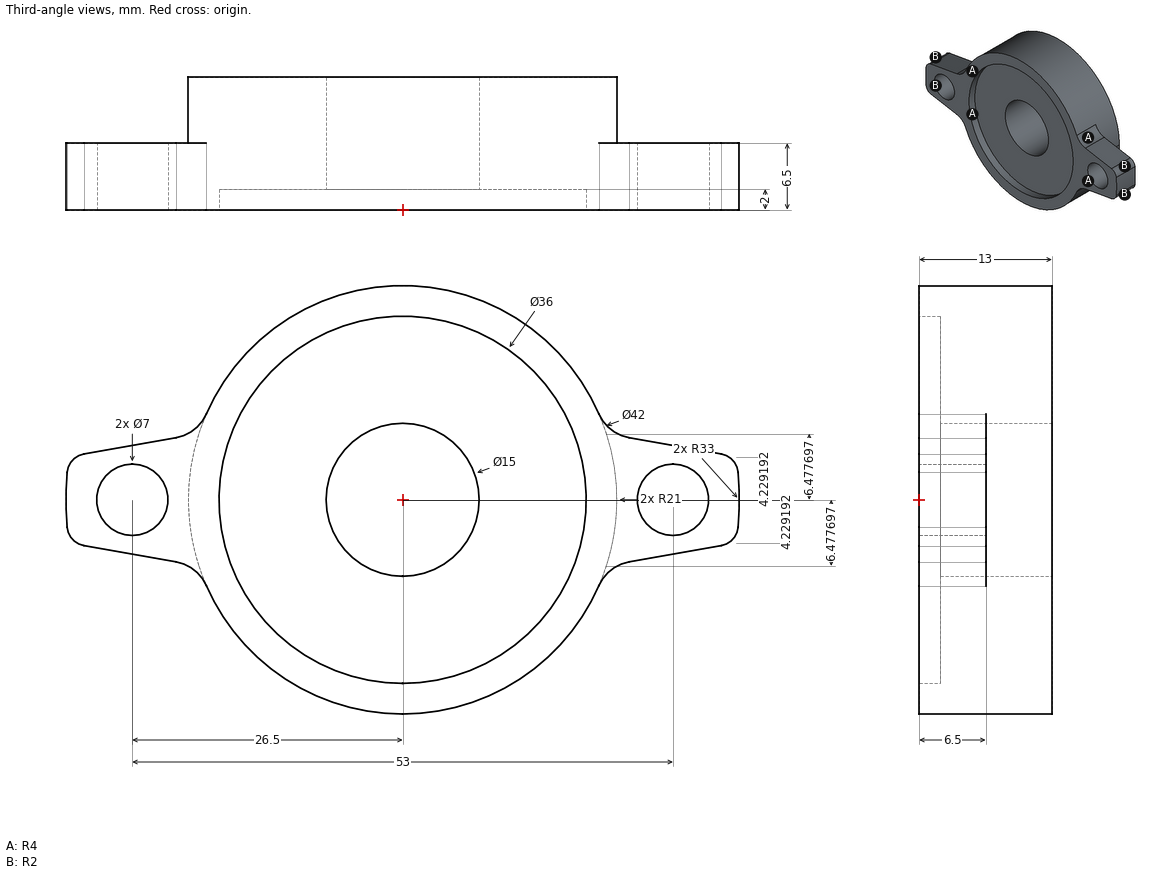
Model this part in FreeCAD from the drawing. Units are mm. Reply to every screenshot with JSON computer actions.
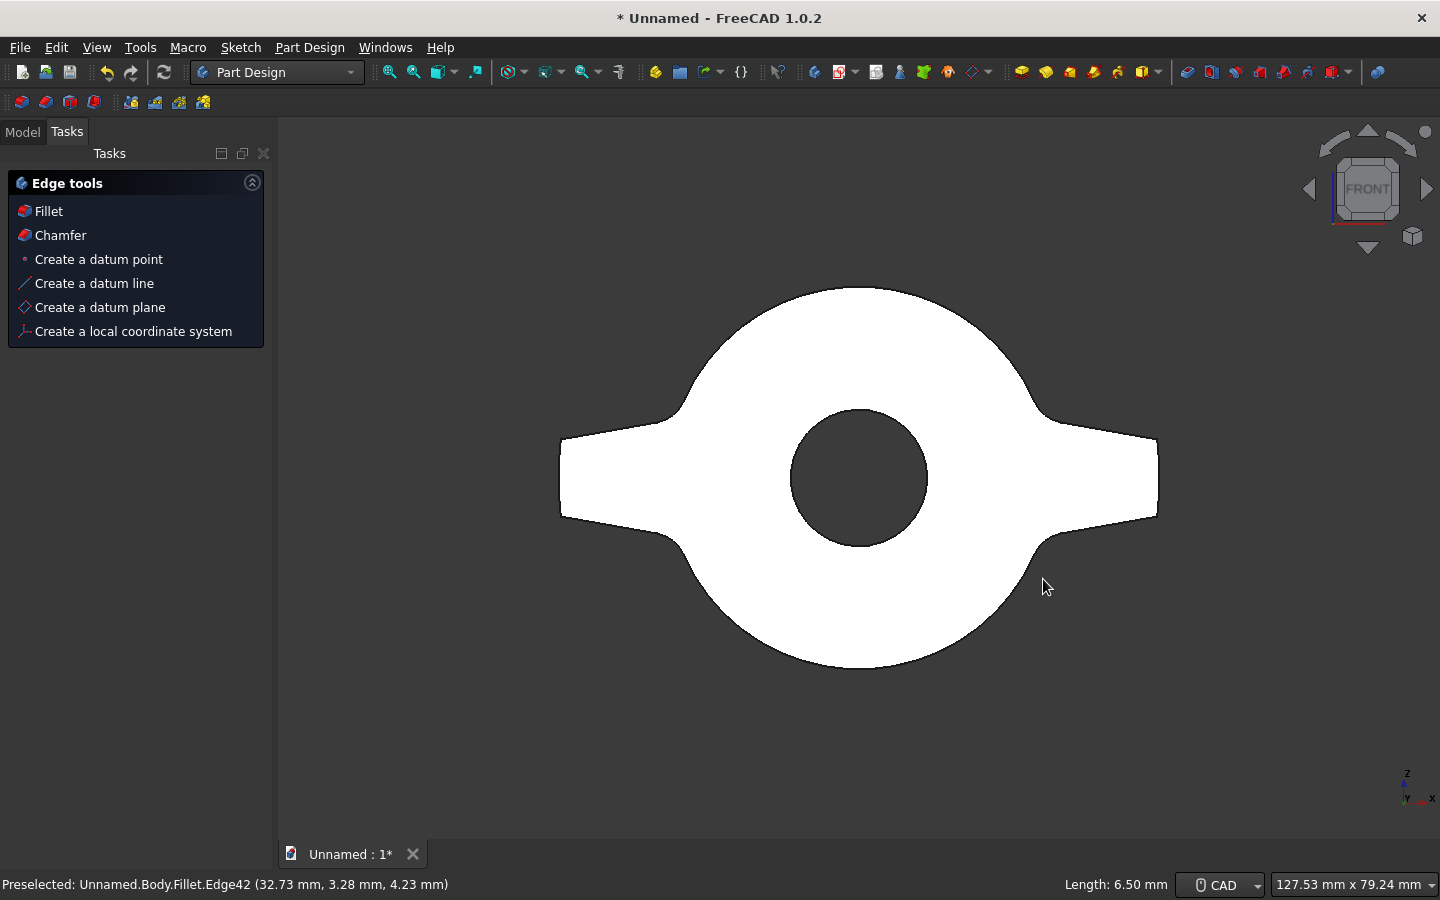
{"action": "key", "text": "3"}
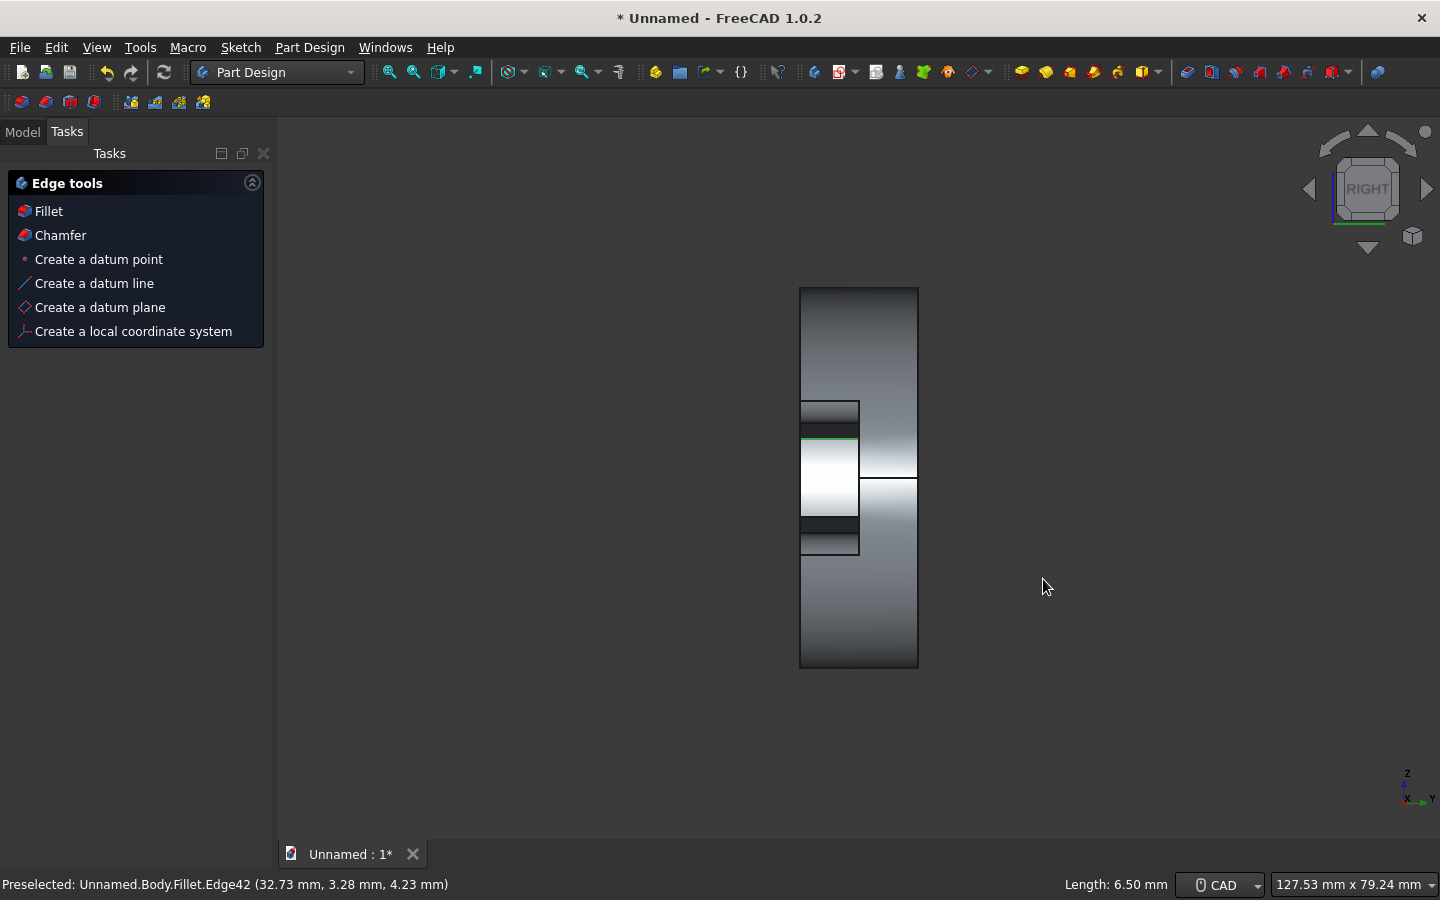
{"action": "key", "text": "5"}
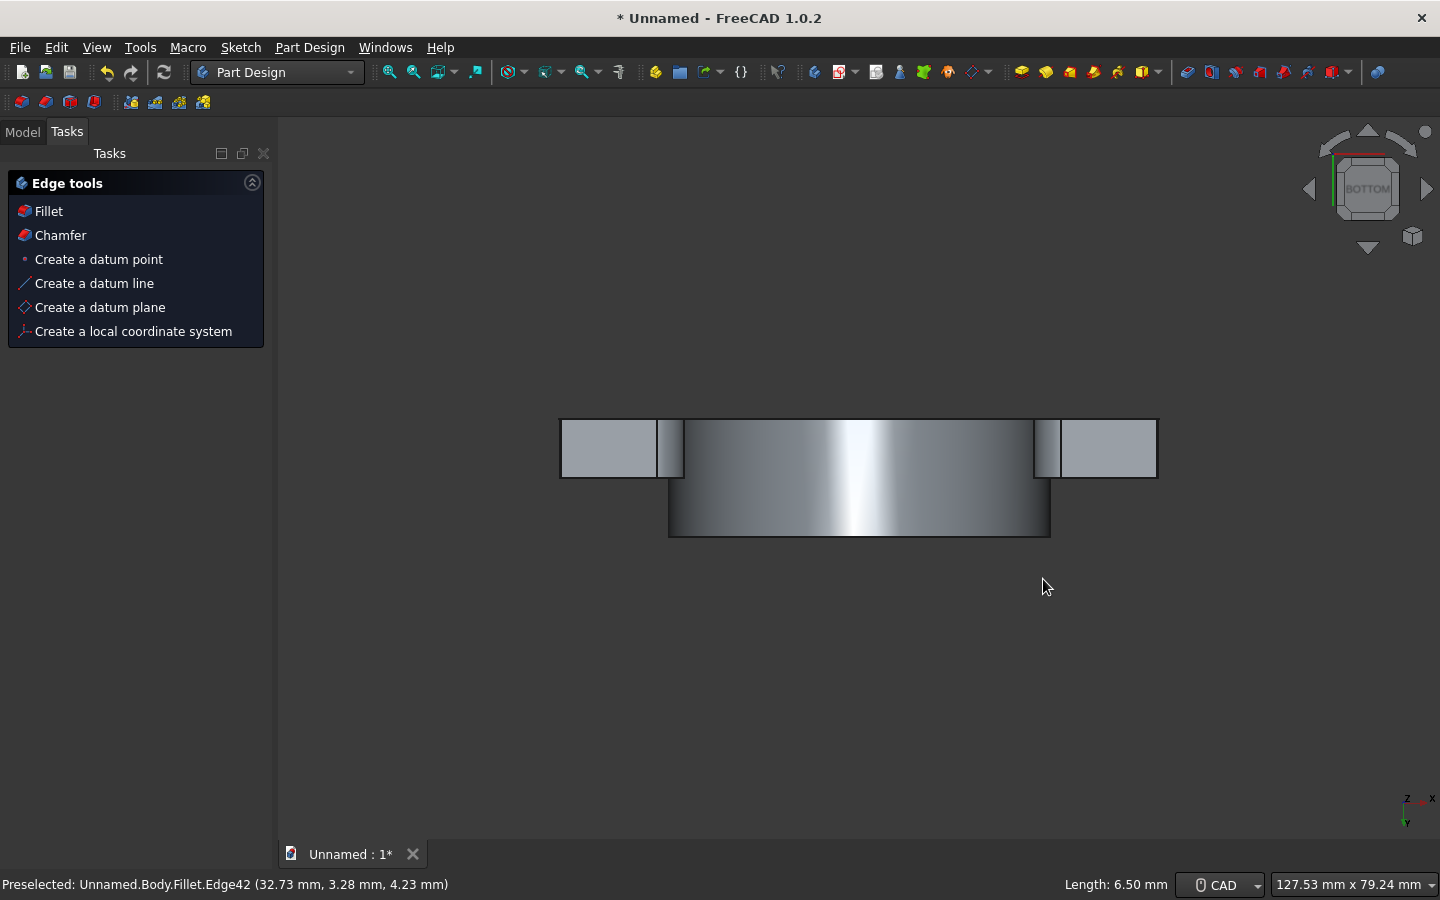
{"action": "key", "text": "4"}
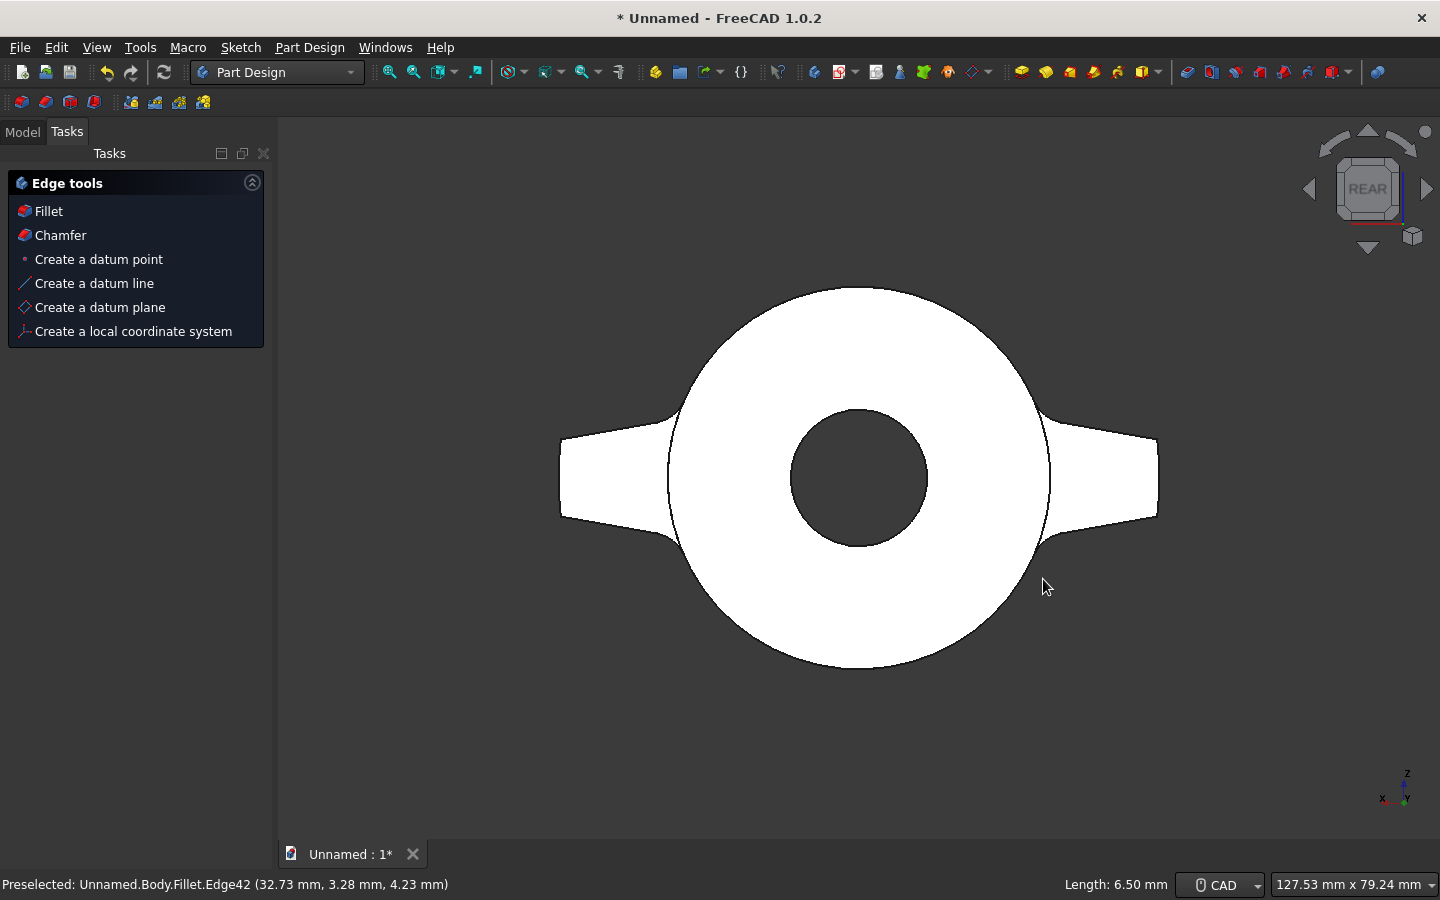
{"action": "key", "text": "6"}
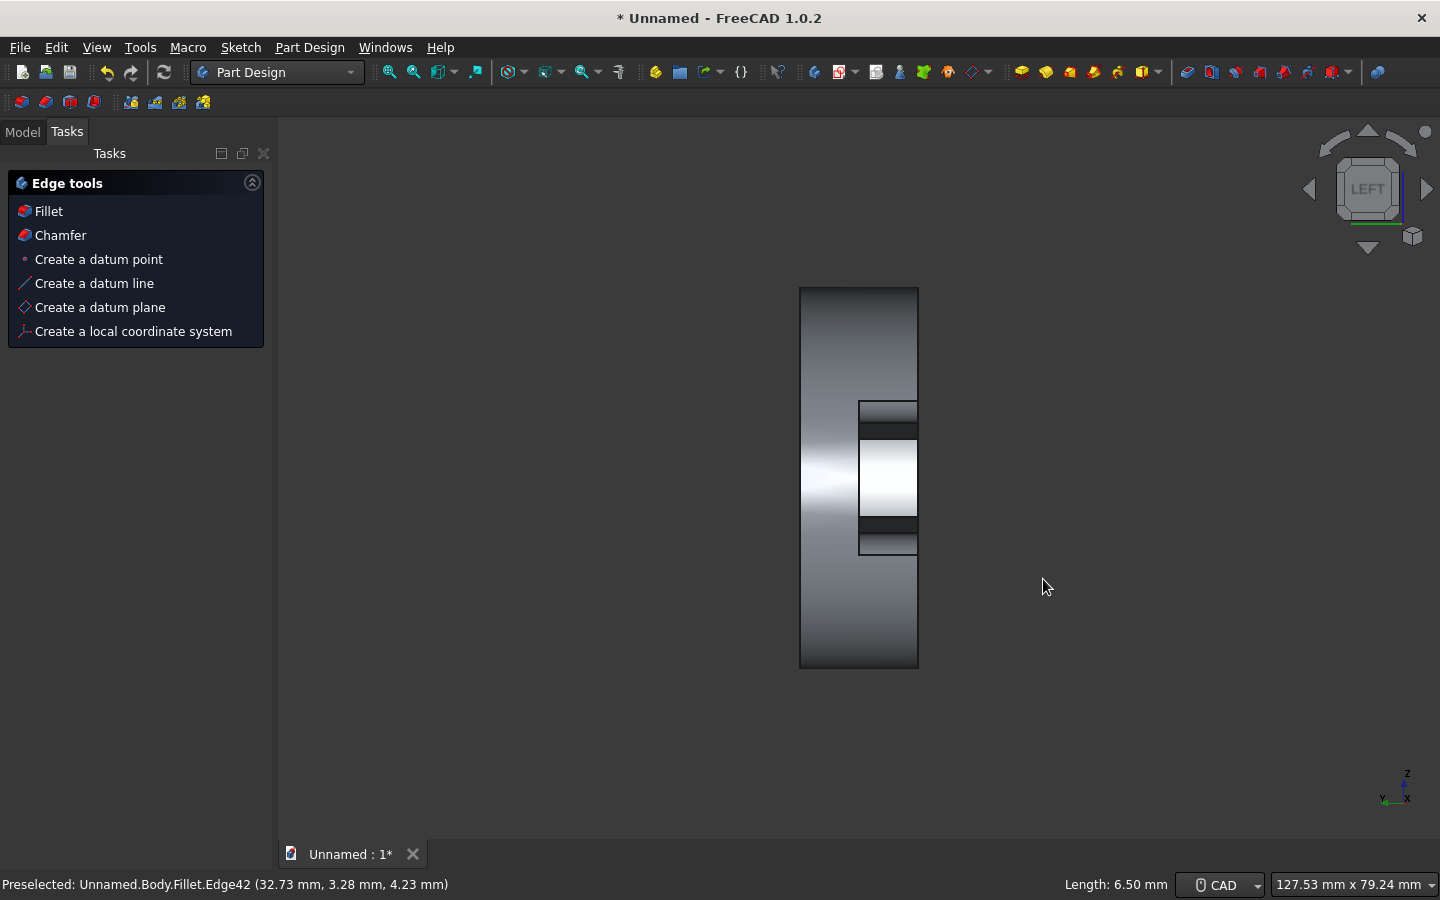
{"action": "key", "text": "v 3"}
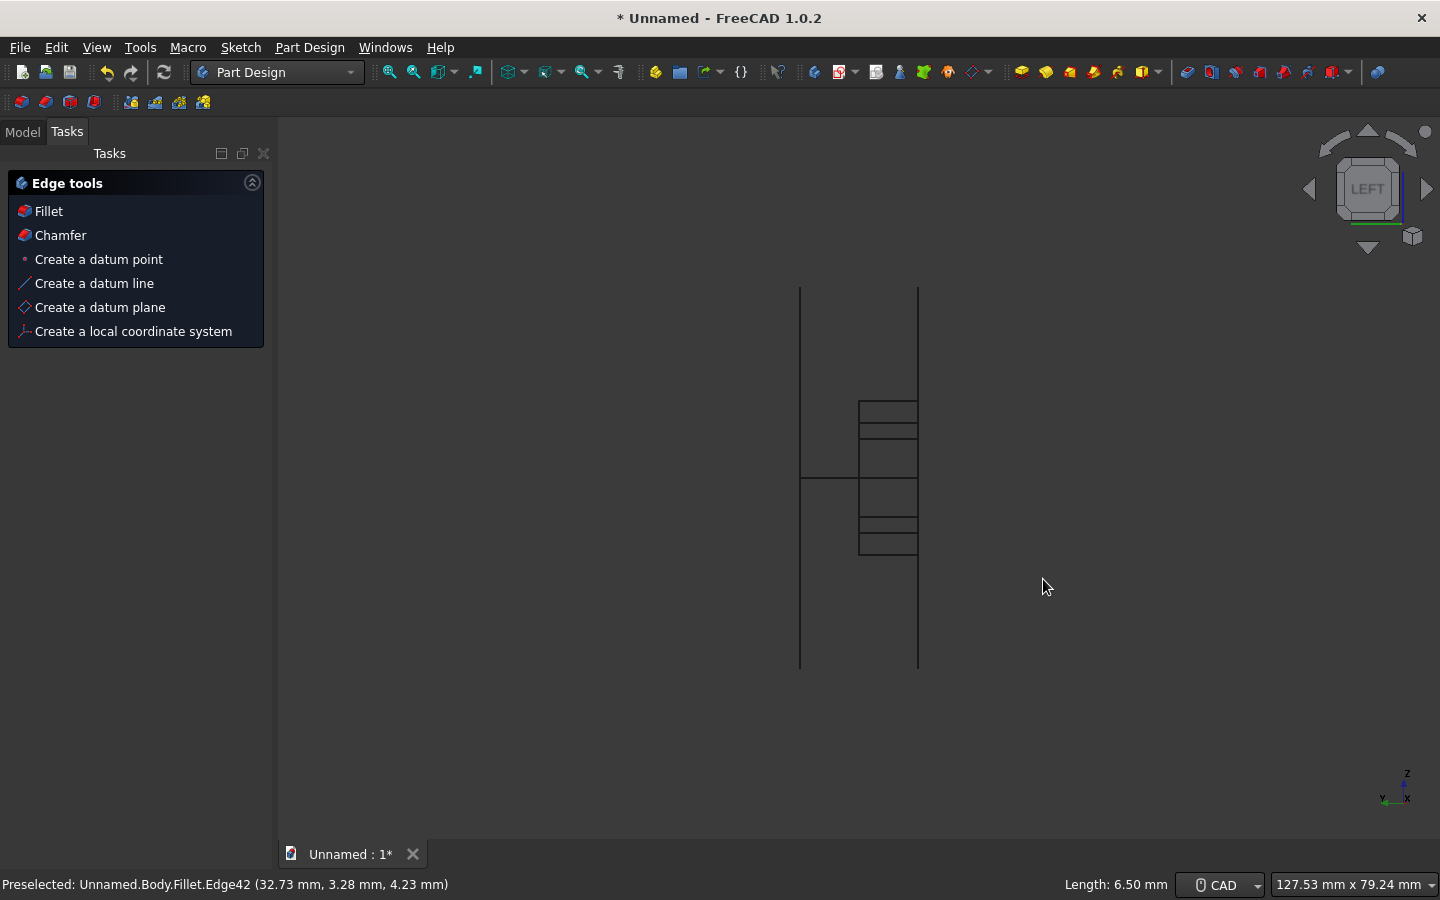
{"action": "key", "text": "0"}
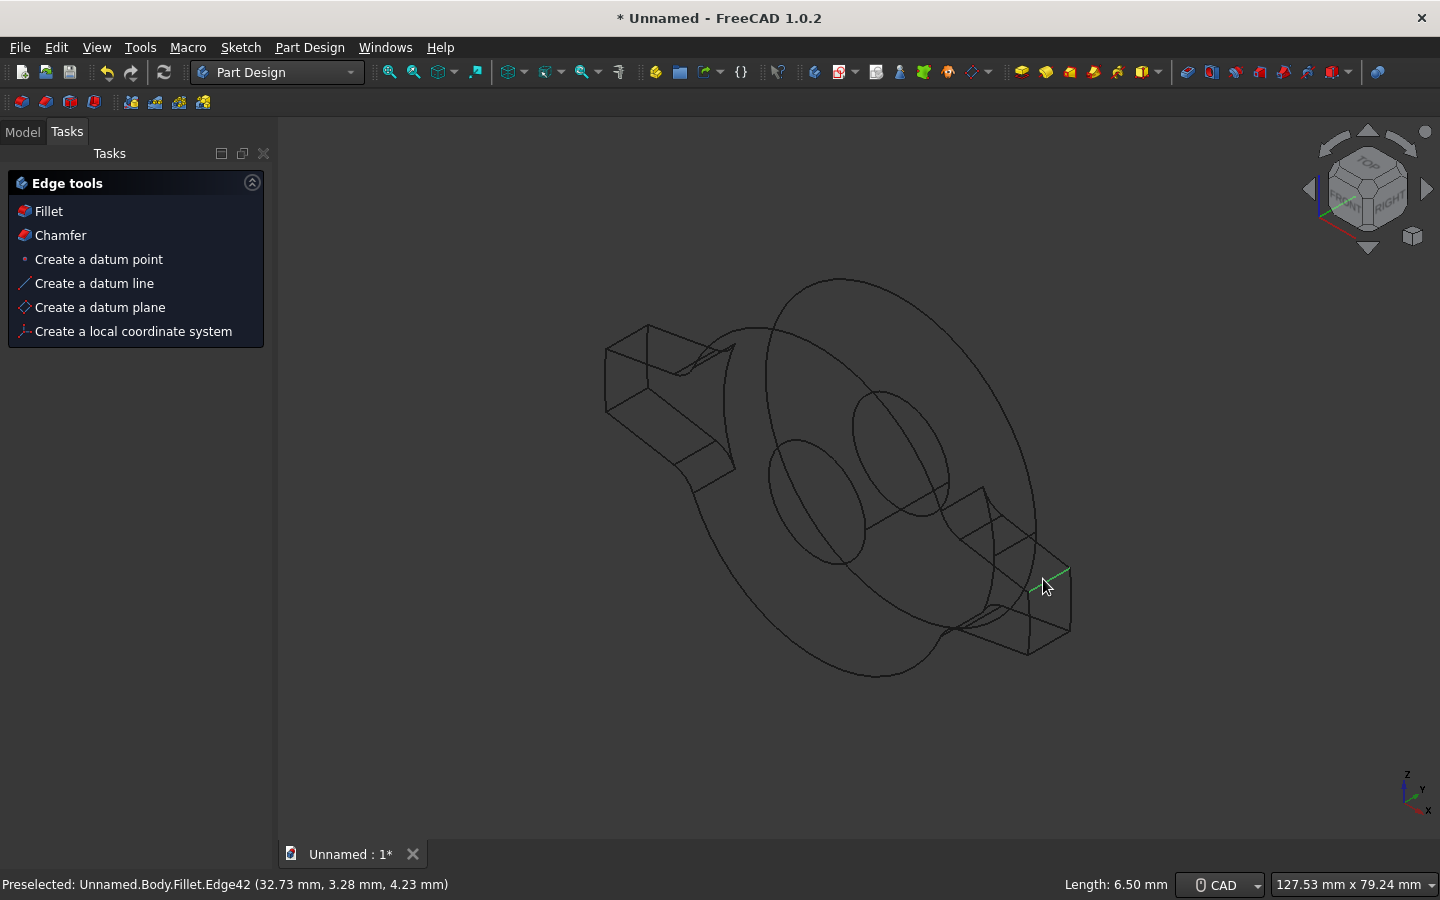
{"action": "left_click", "coordinate": [1049, 642], "text": "ctrl"}